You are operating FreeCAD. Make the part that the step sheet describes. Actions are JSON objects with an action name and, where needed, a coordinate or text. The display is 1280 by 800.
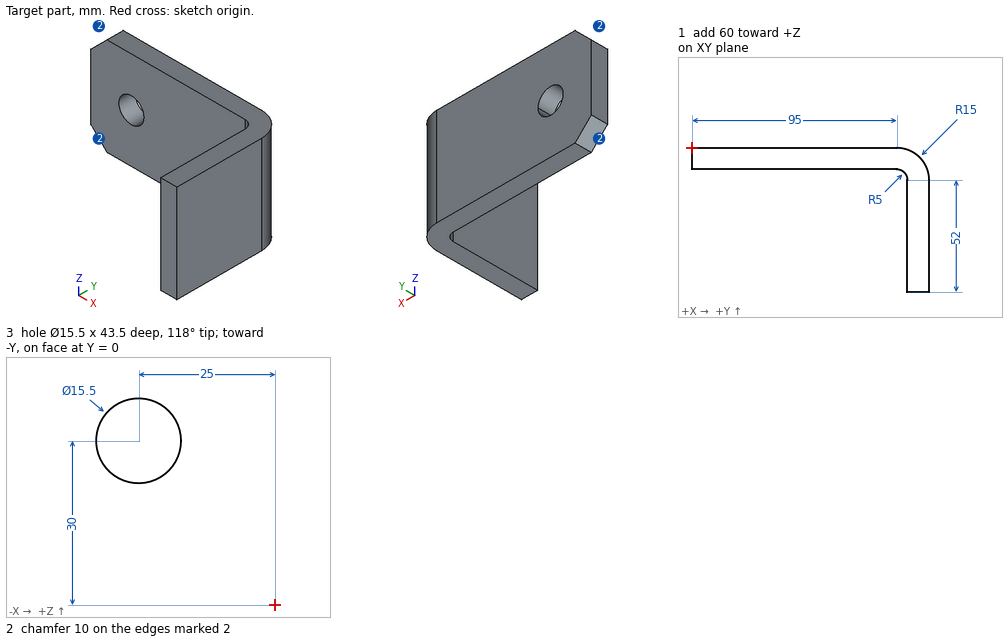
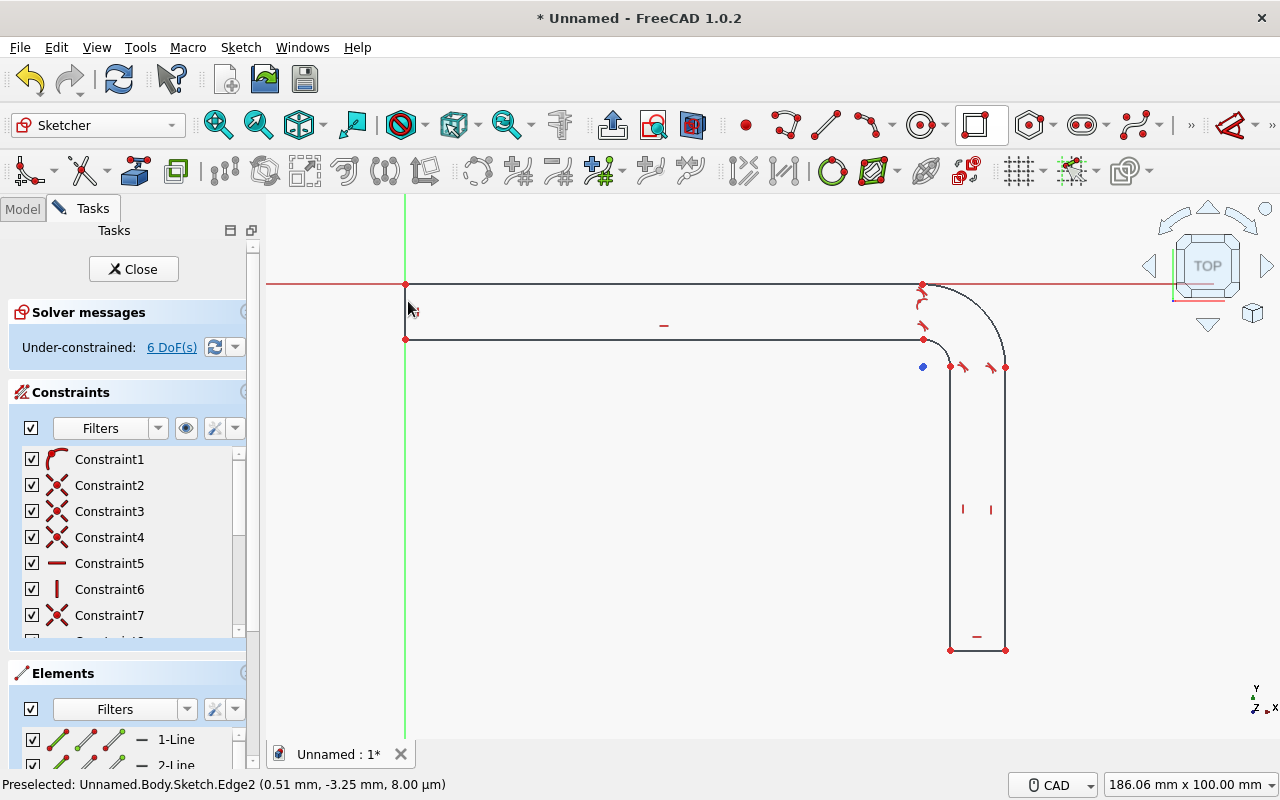
{"action": "left_click", "coordinate": [947, 354]}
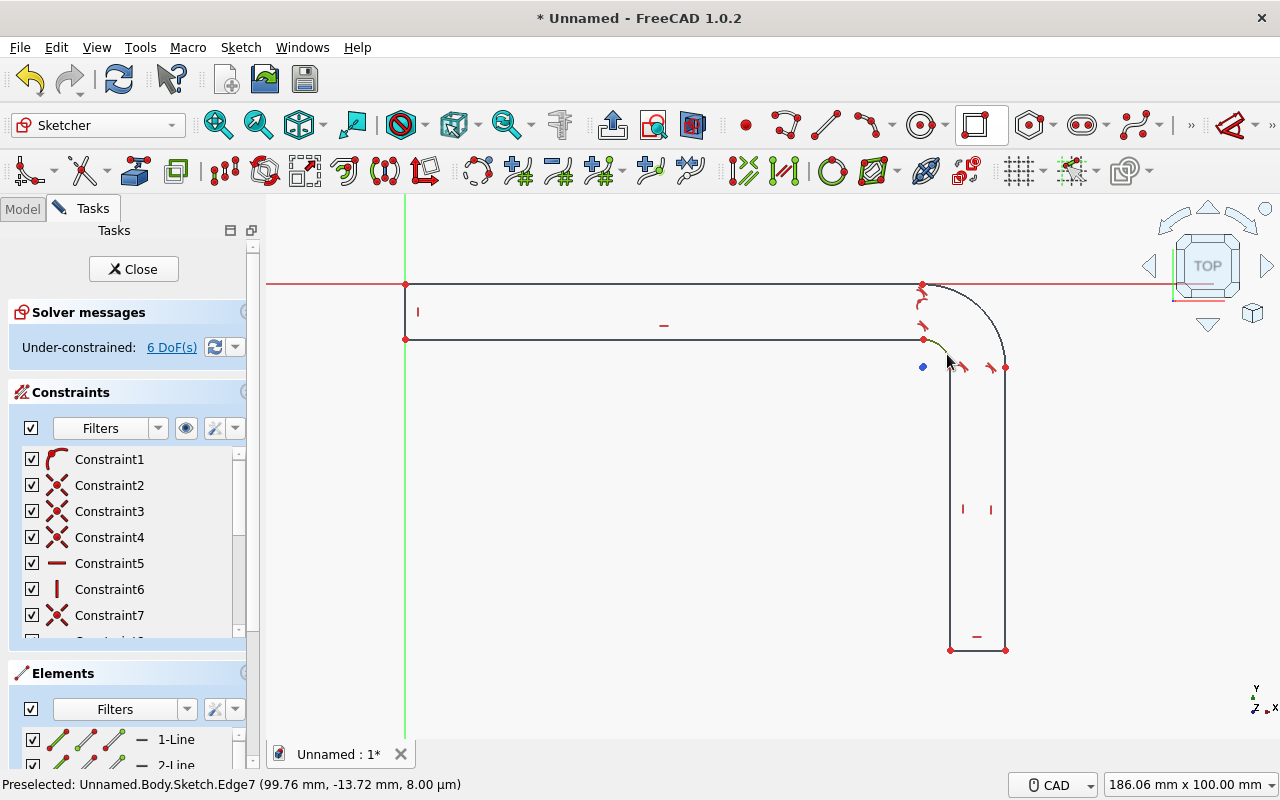
{"action": "left_click", "coordinate": [996, 330]}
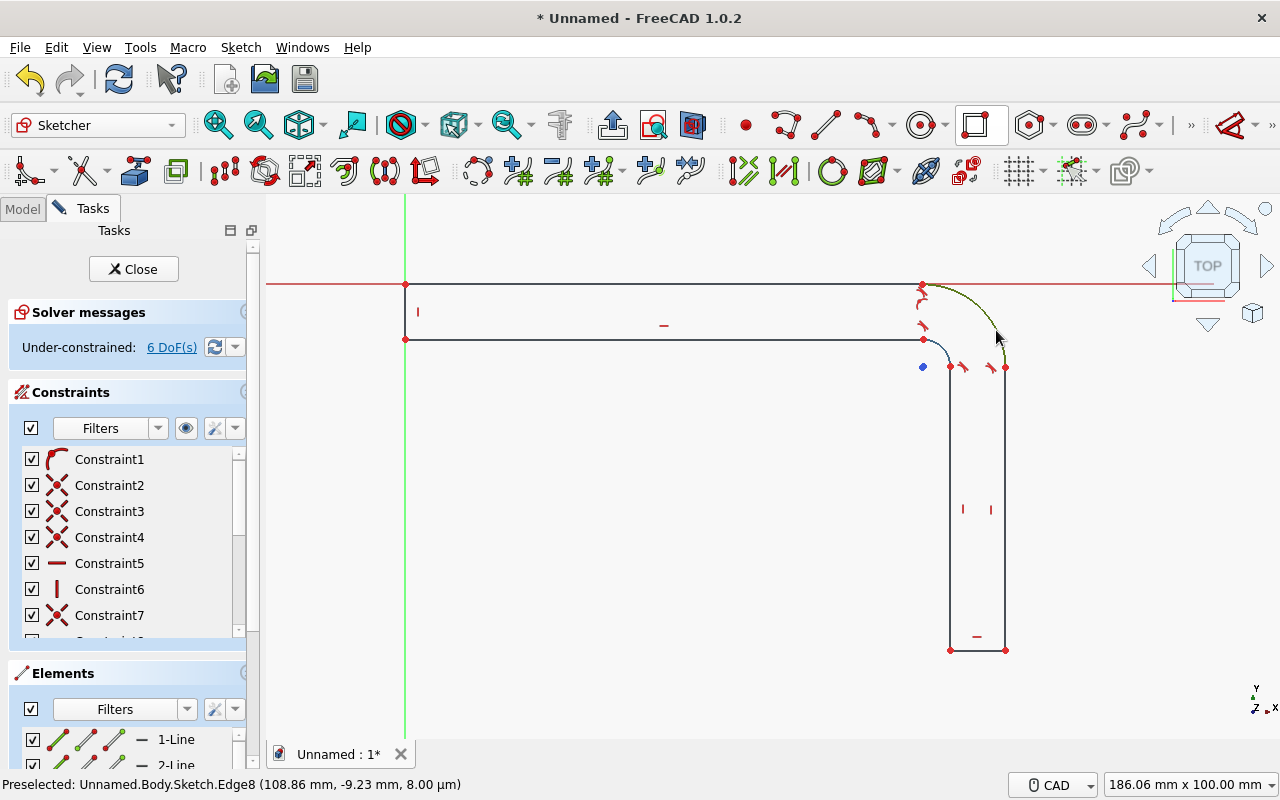
{"action": "key", "text": "c"}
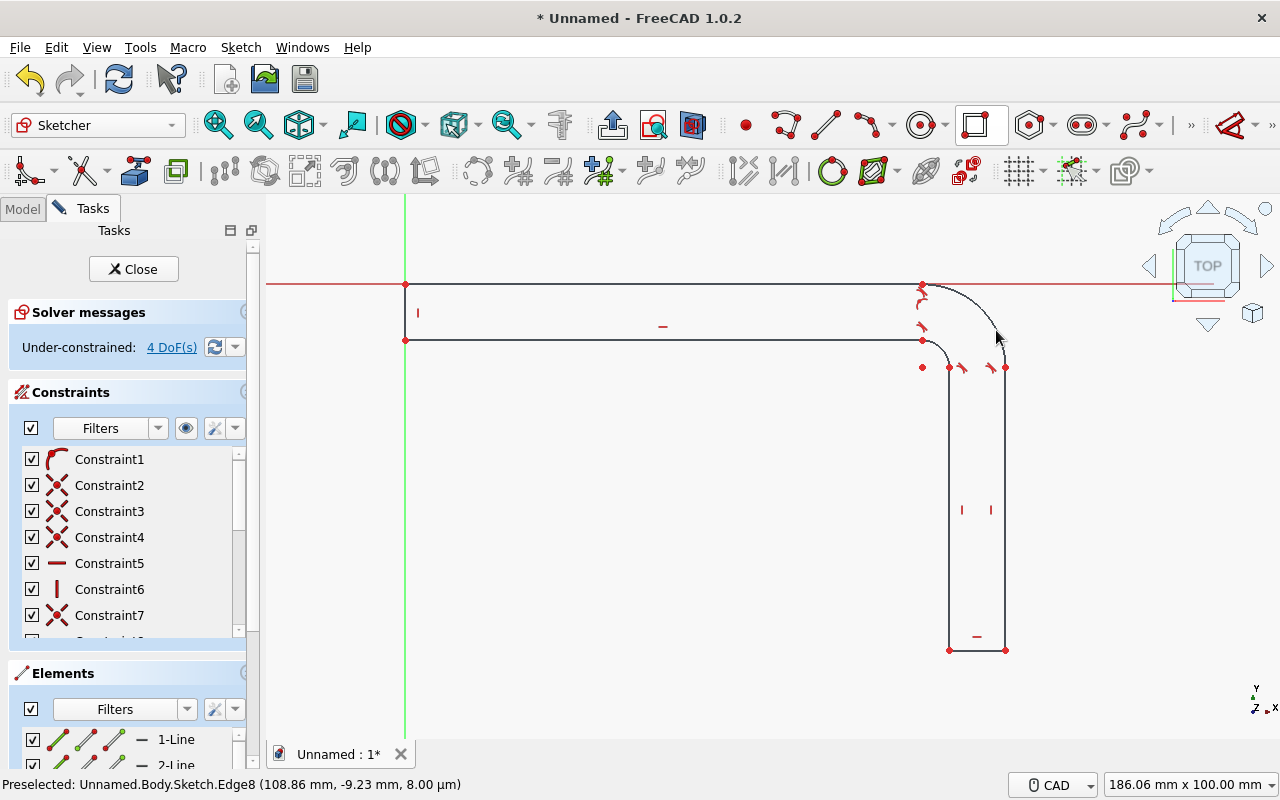
{"action": "left_click", "coordinate": [1230, 126]}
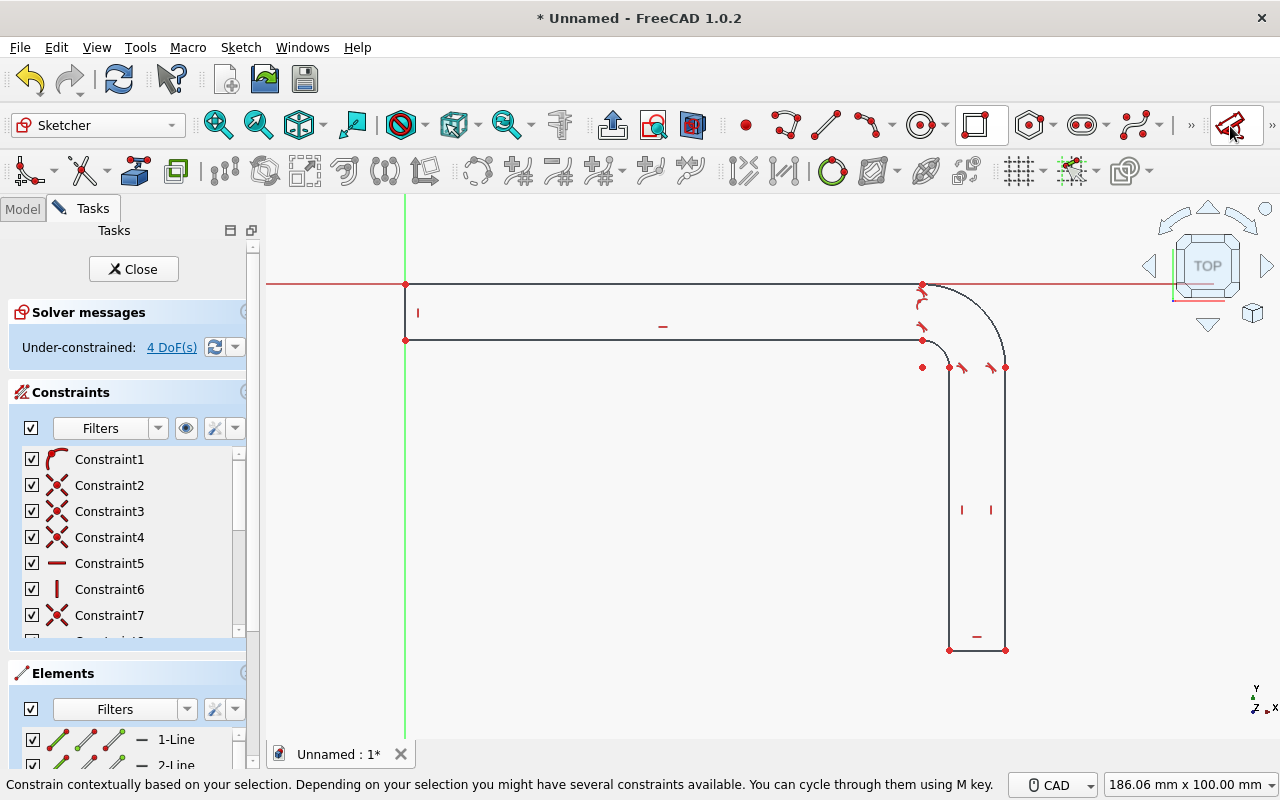
{"action": "scroll", "coordinate": [946, 355], "scroll_direction": "up", "scroll_amount": 2}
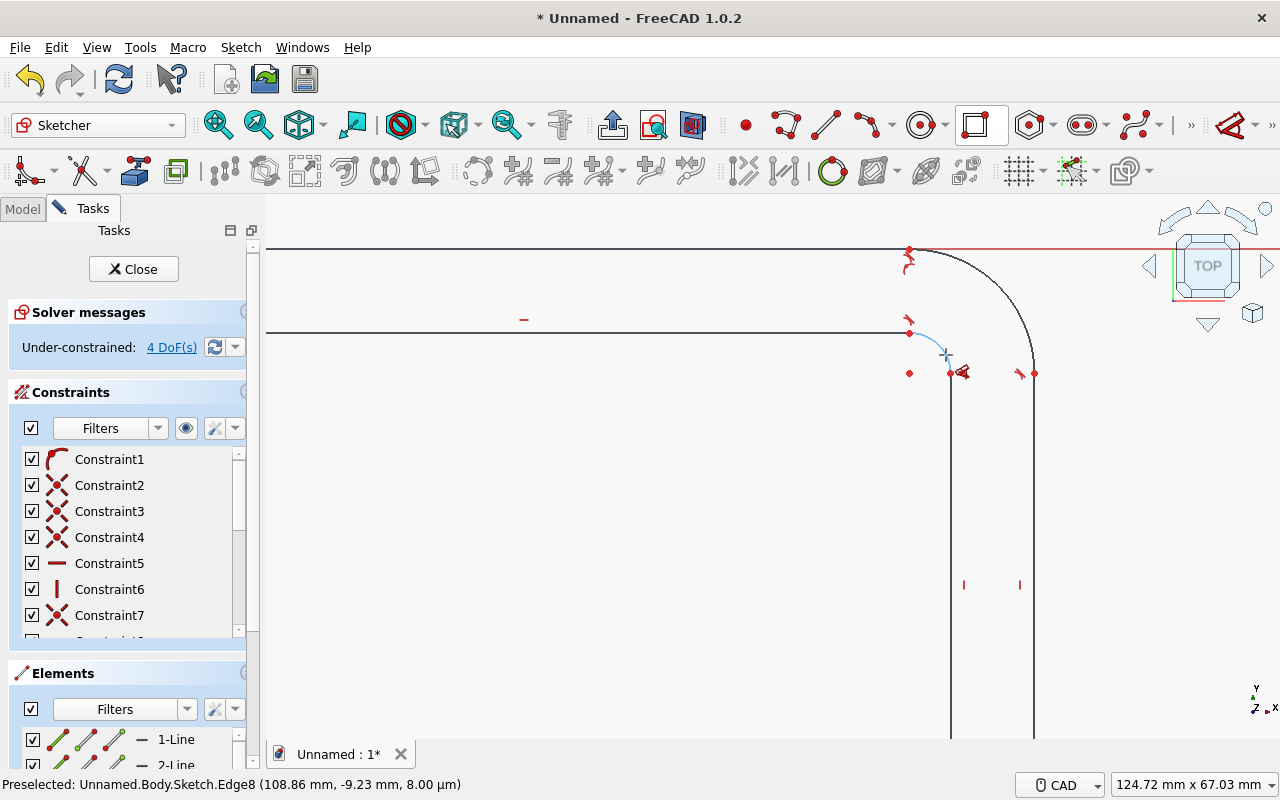
{"action": "left_click", "coordinate": [946, 355]}
{"action": "left_click", "coordinate": [974, 340]}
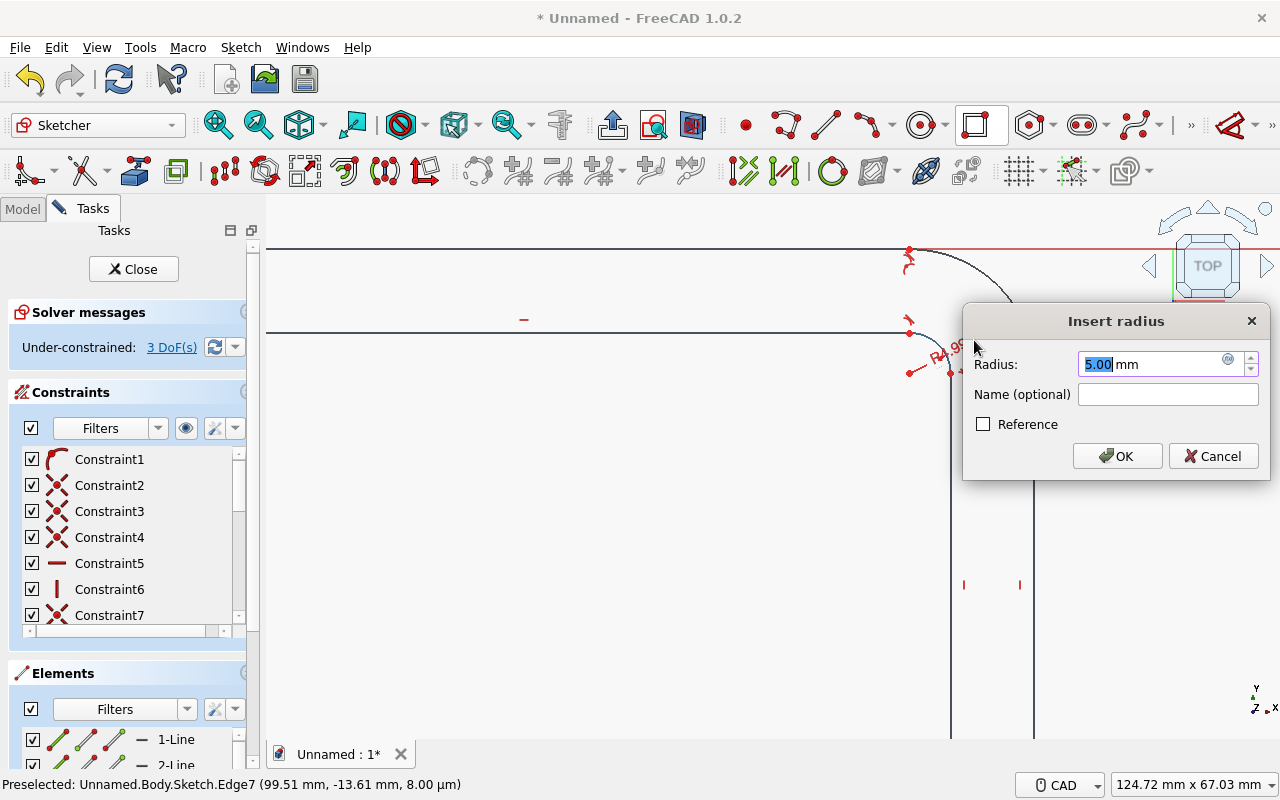
{"action": "type", "text": "5"}
{"action": "key", "text": "Return"}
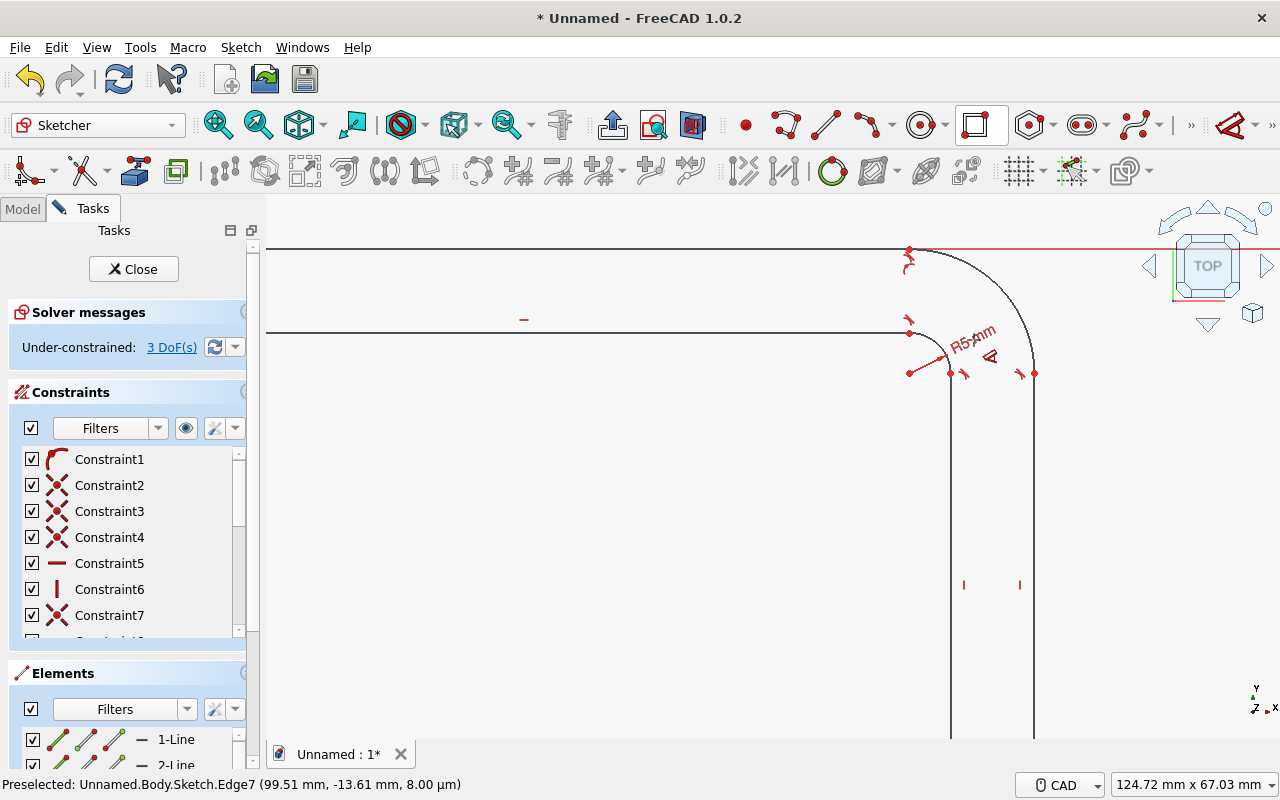
{"action": "left_click", "coordinate": [1021, 317]}
{"action": "left_click", "coordinate": [1049, 302]}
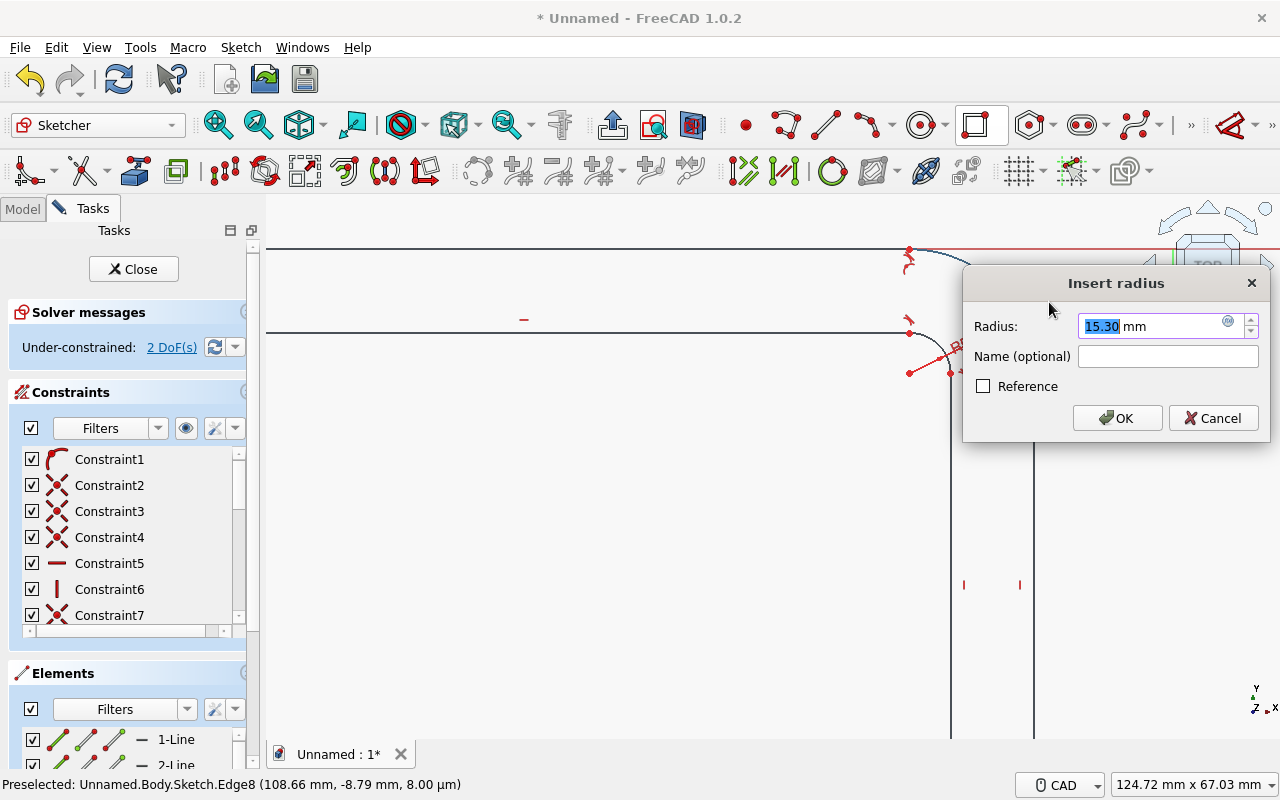
{"action": "type", "text": "15"}
{"action": "key", "text": "Return"}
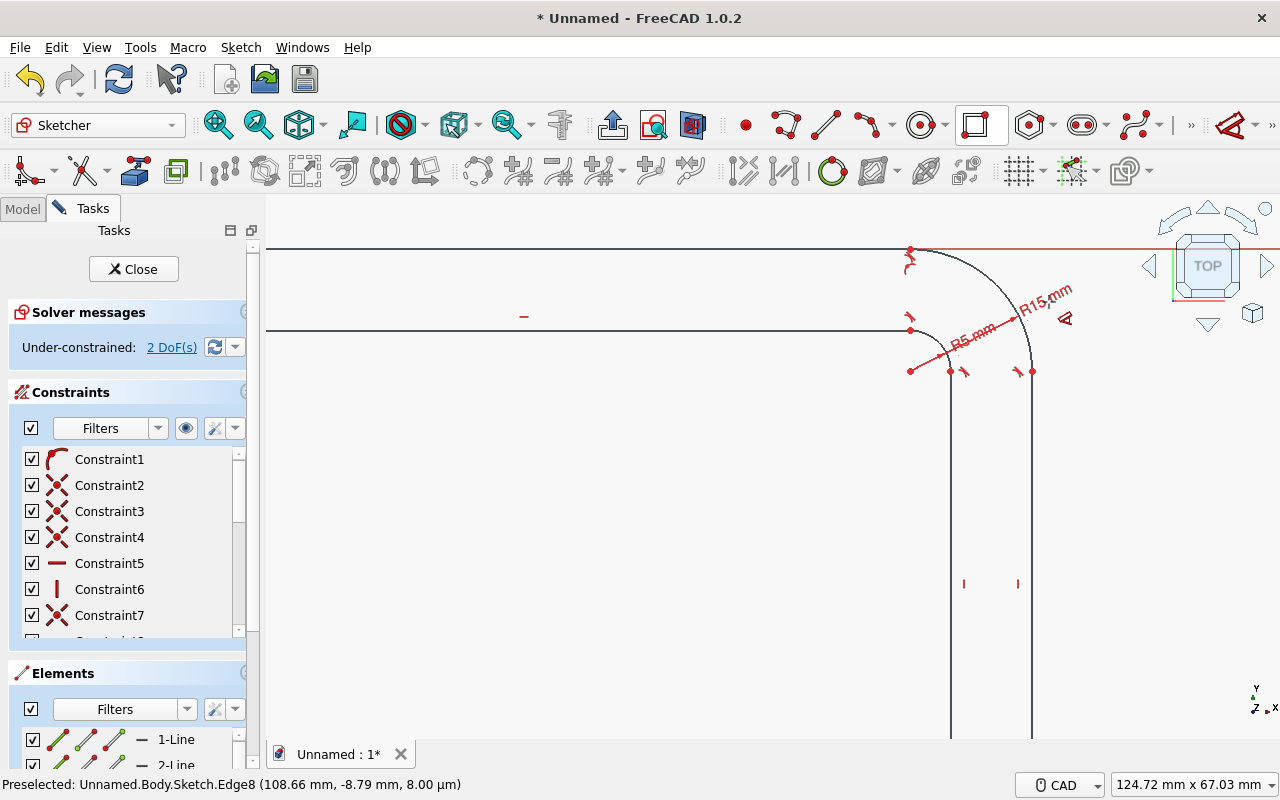
{"action": "left_click", "coordinate": [679, 249]}
{"action": "left_click", "coordinate": [602, 283]}